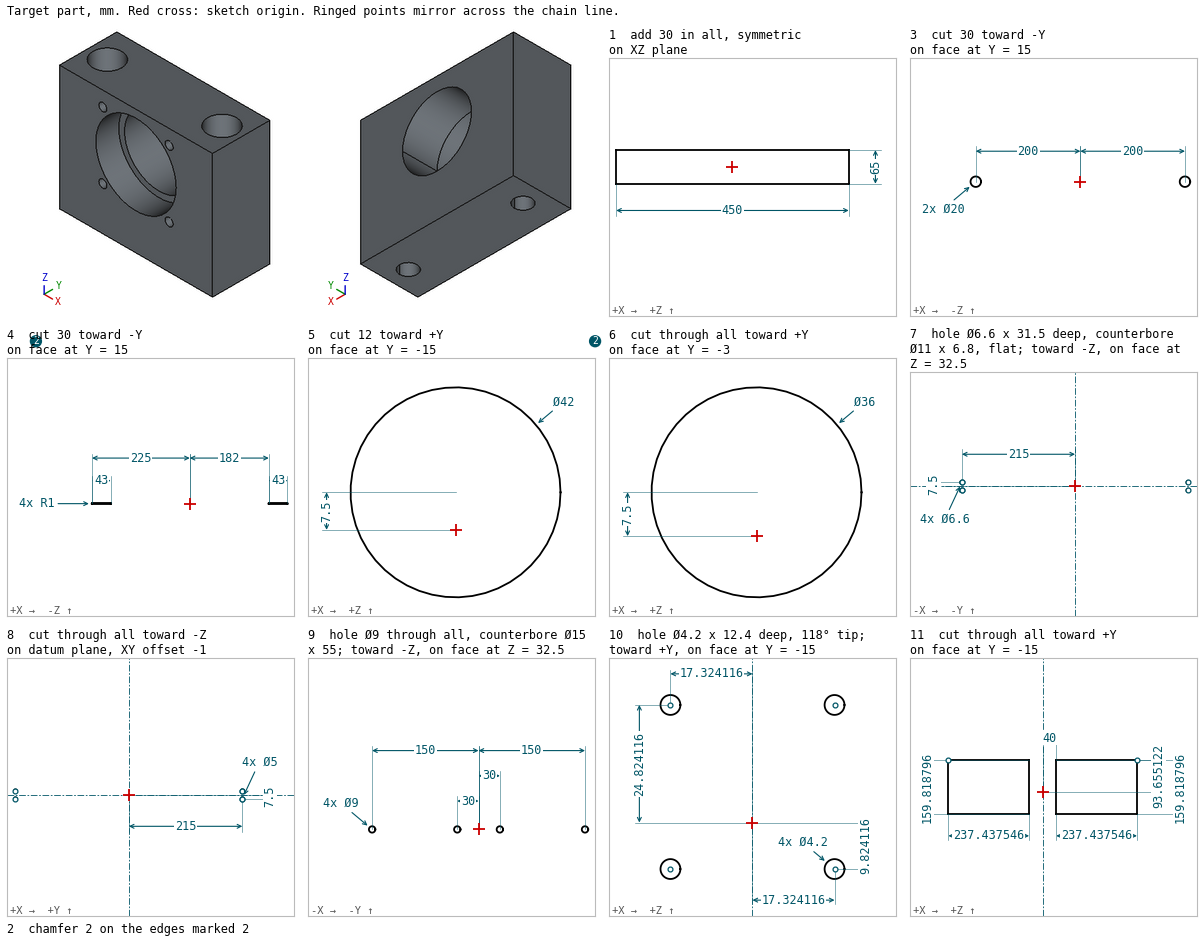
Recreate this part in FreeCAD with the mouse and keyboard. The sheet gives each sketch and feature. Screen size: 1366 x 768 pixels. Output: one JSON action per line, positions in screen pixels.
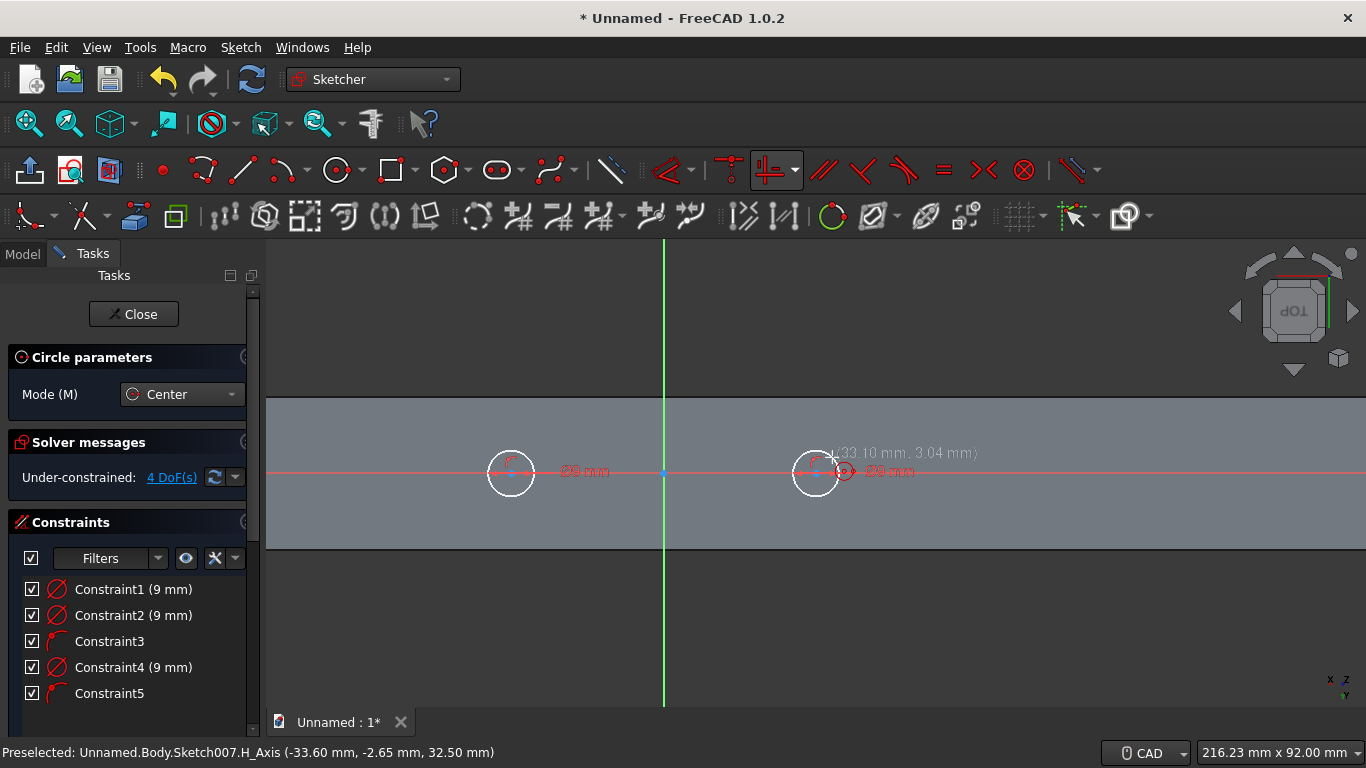
{"action": "scroll", "coordinate": [816, 473], "scroll_direction": "down", "scroll_amount": 4}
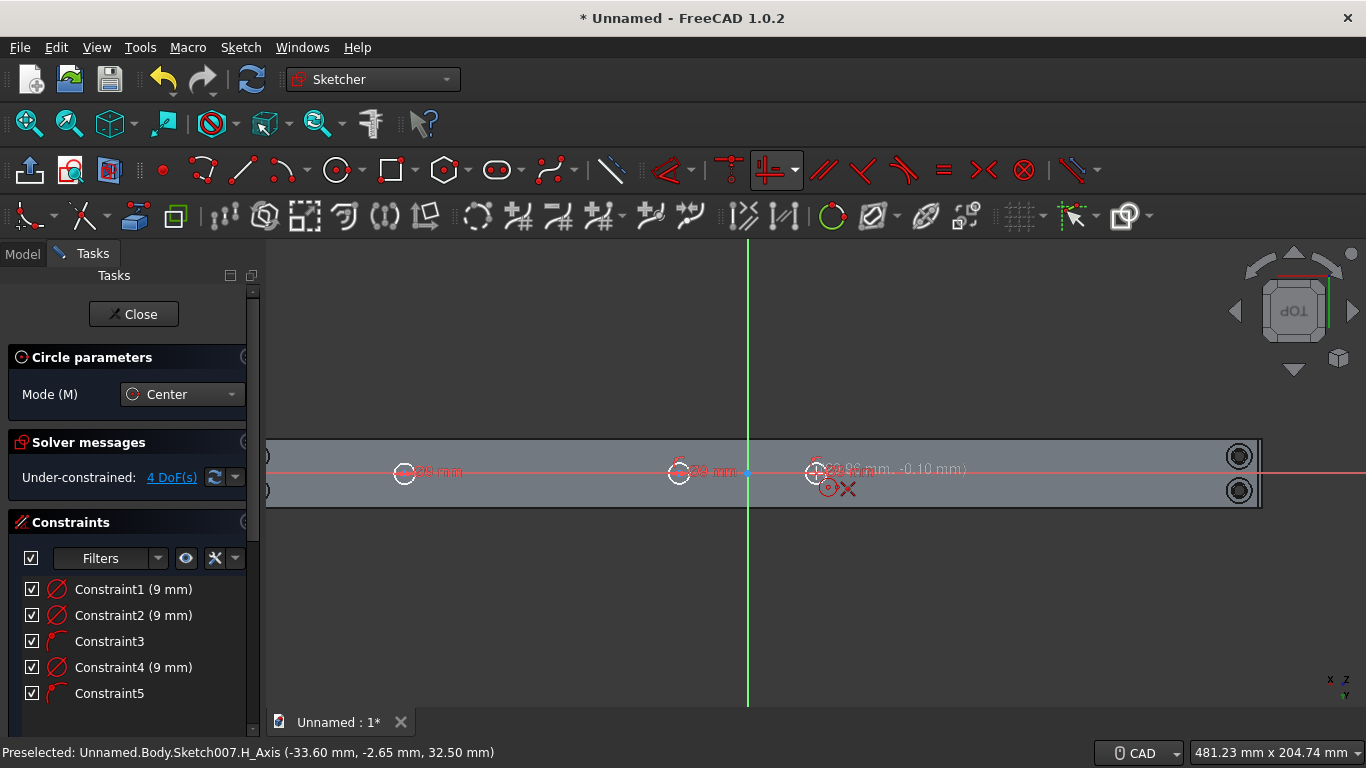
{"action": "scroll", "coordinate": [1091, 473], "scroll_direction": "up", "scroll_amount": 4}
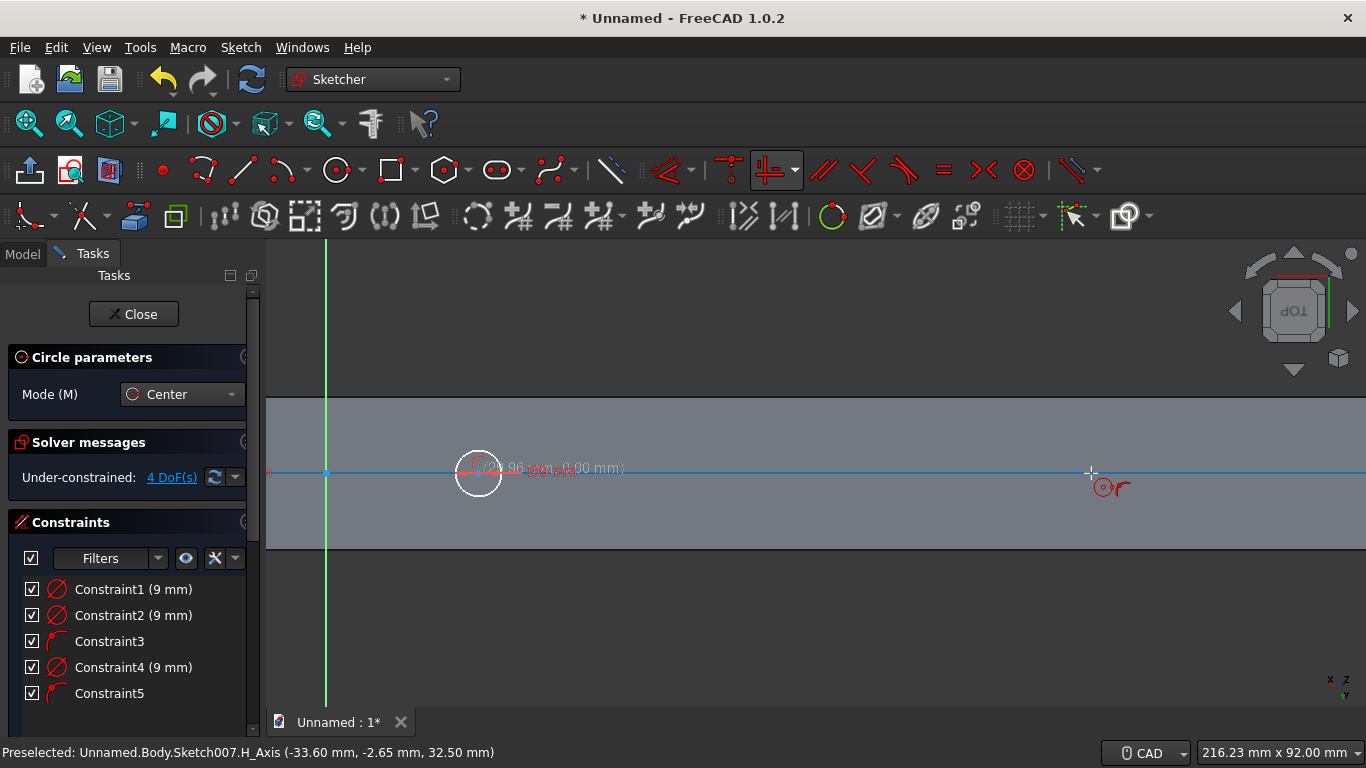
{"action": "left_click", "coordinate": [1089, 473]}
{"action": "mouse_move", "coordinate": [1106, 457]}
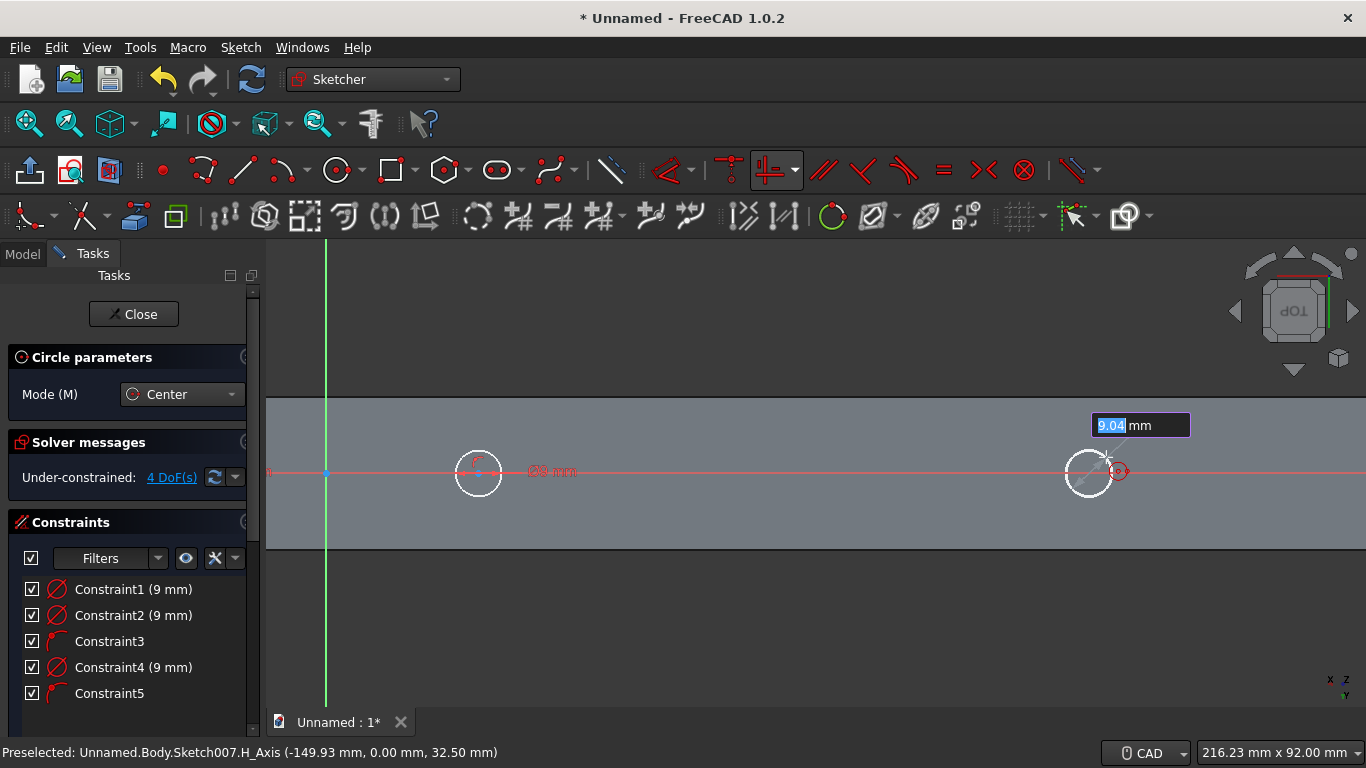
{"action": "type", "text": "9"}
{"action": "key", "text": "Return"}
{"action": "key", "text": "Escape"}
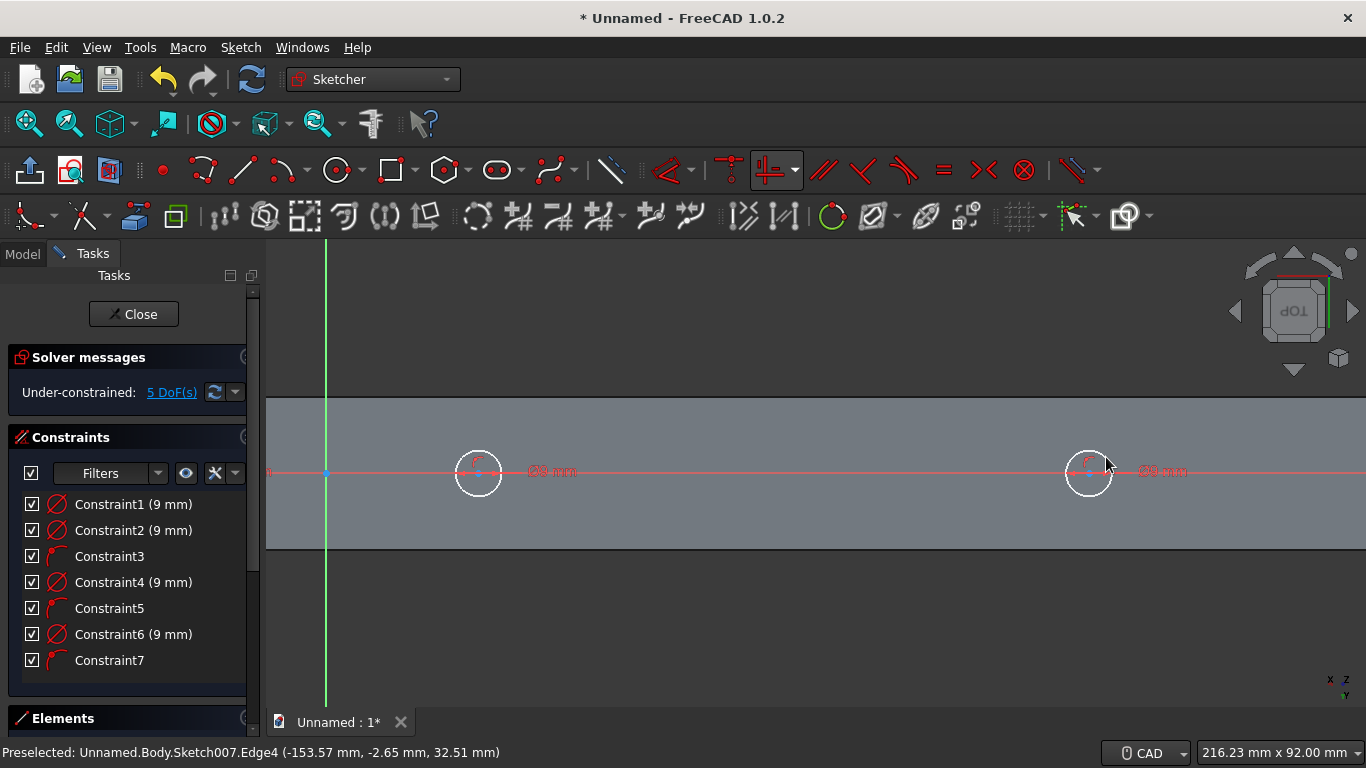
{"action": "scroll", "coordinate": [1091, 473], "scroll_direction": "down", "scroll_amount": 4}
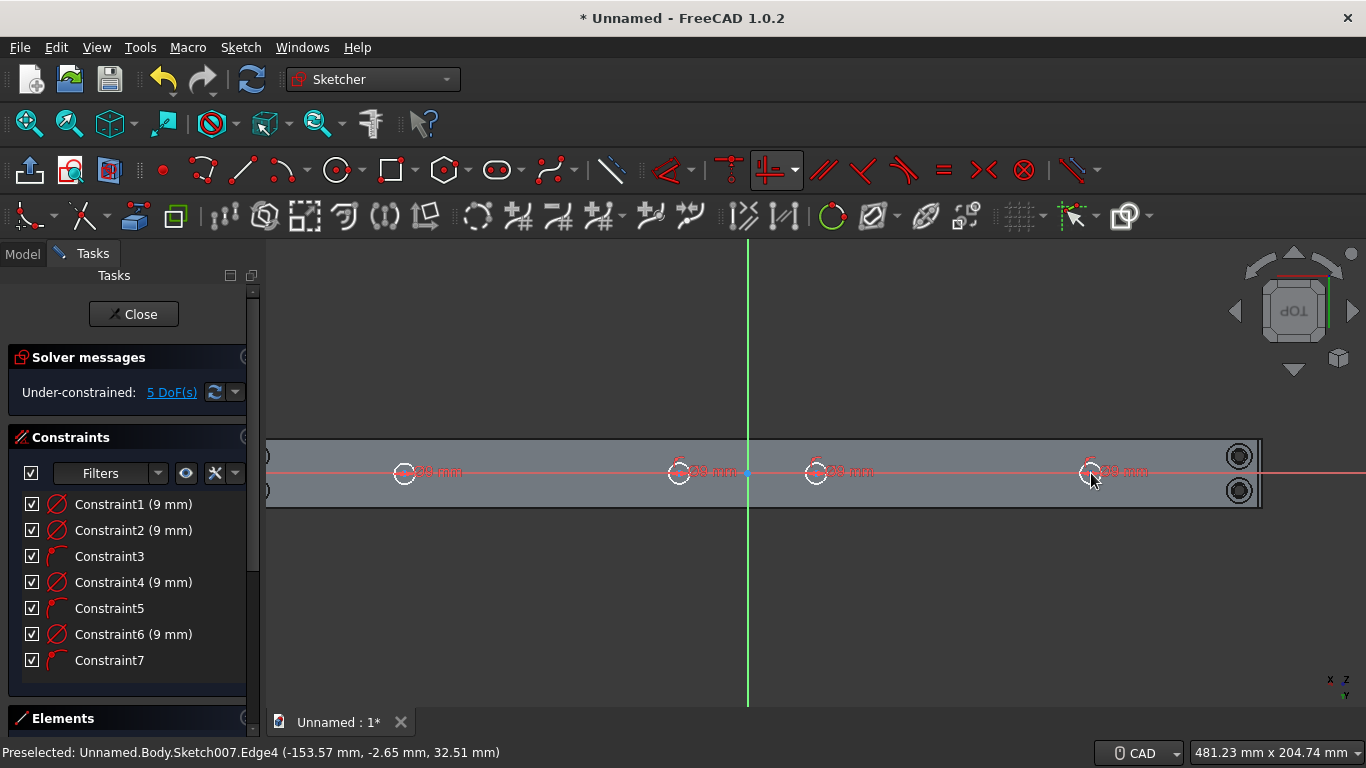
{"action": "left_click", "coordinate": [405, 474]}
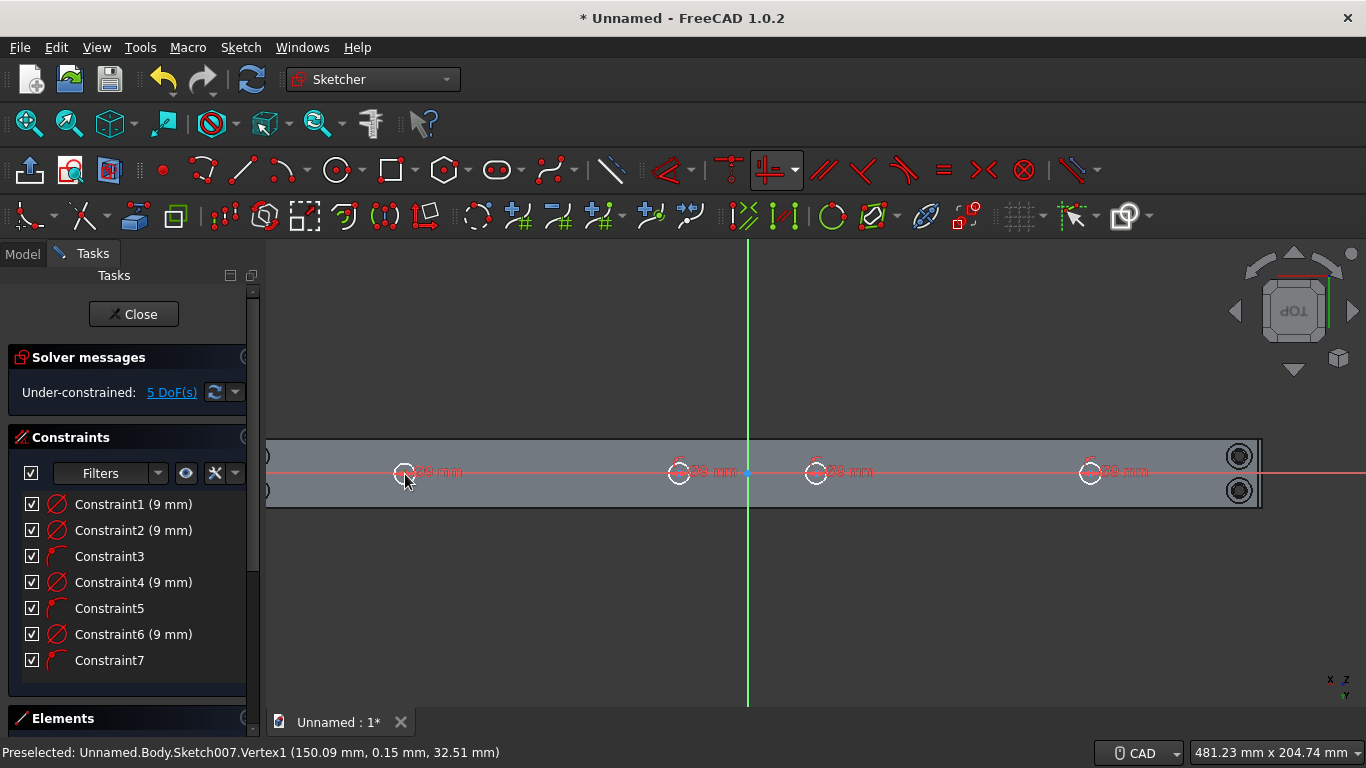
{"action": "left_click", "coordinate": [359, 473]}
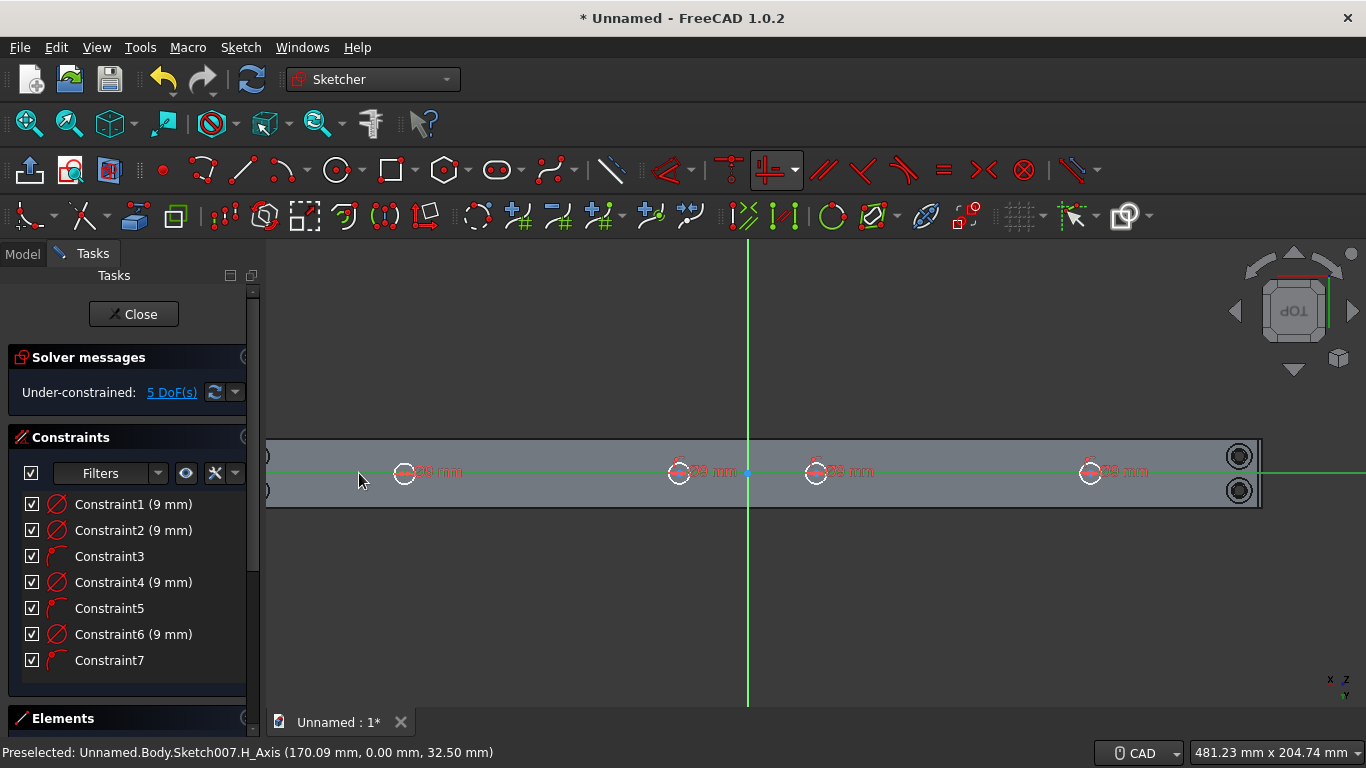
{"action": "key", "text": "c"}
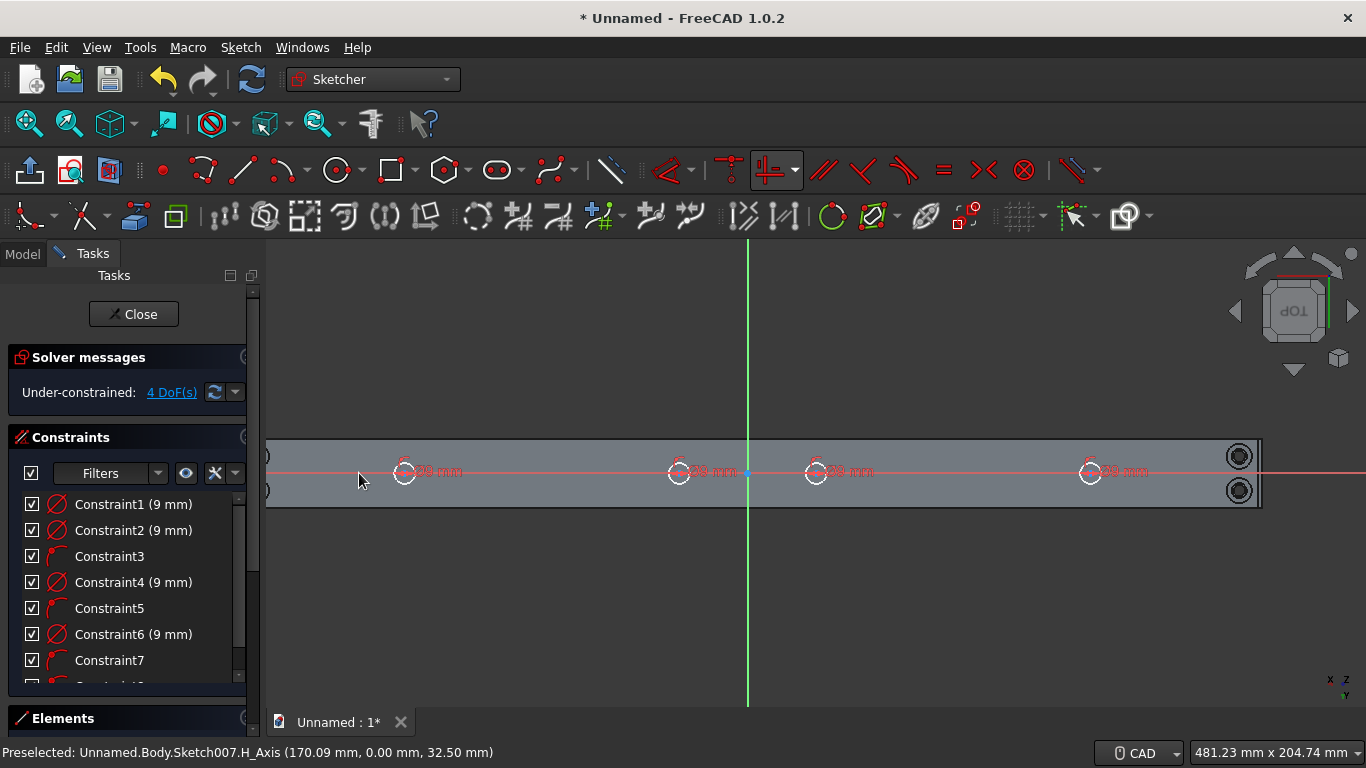
{"action": "key", "text": "d"}